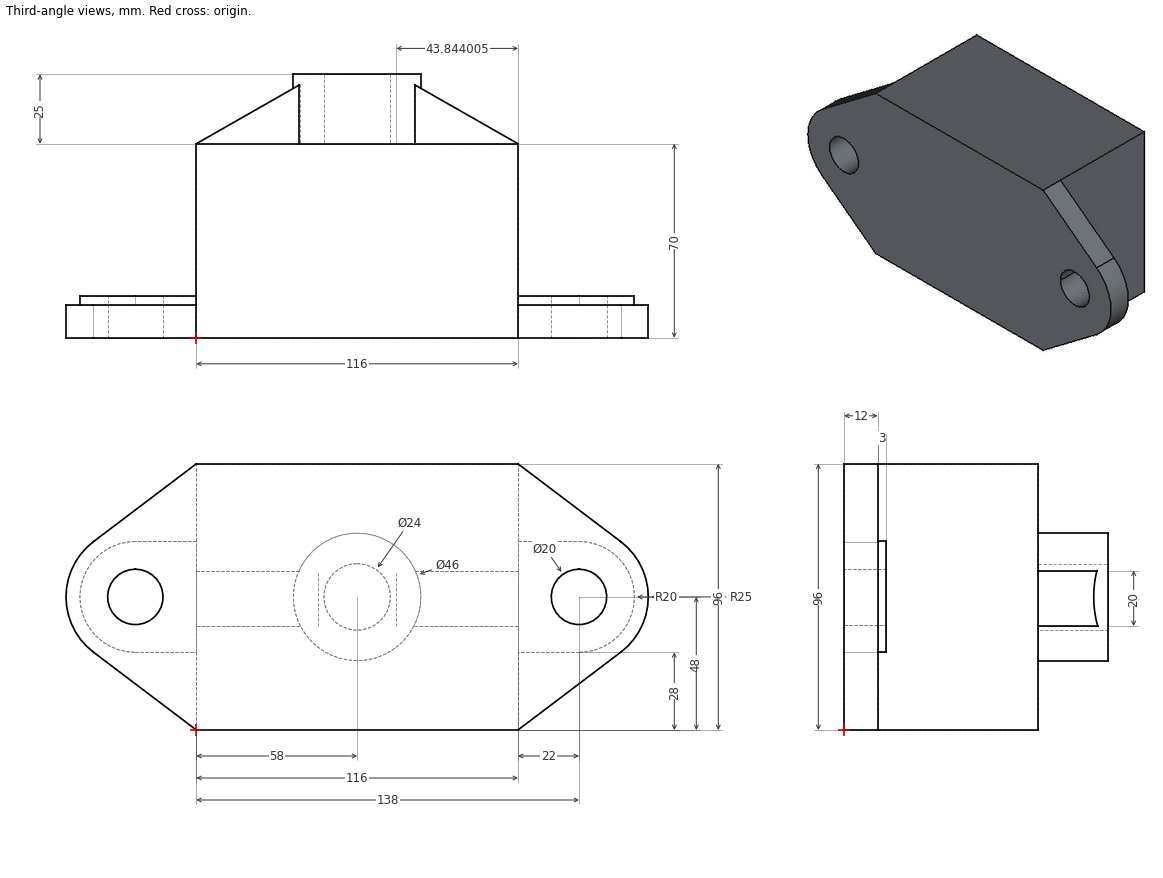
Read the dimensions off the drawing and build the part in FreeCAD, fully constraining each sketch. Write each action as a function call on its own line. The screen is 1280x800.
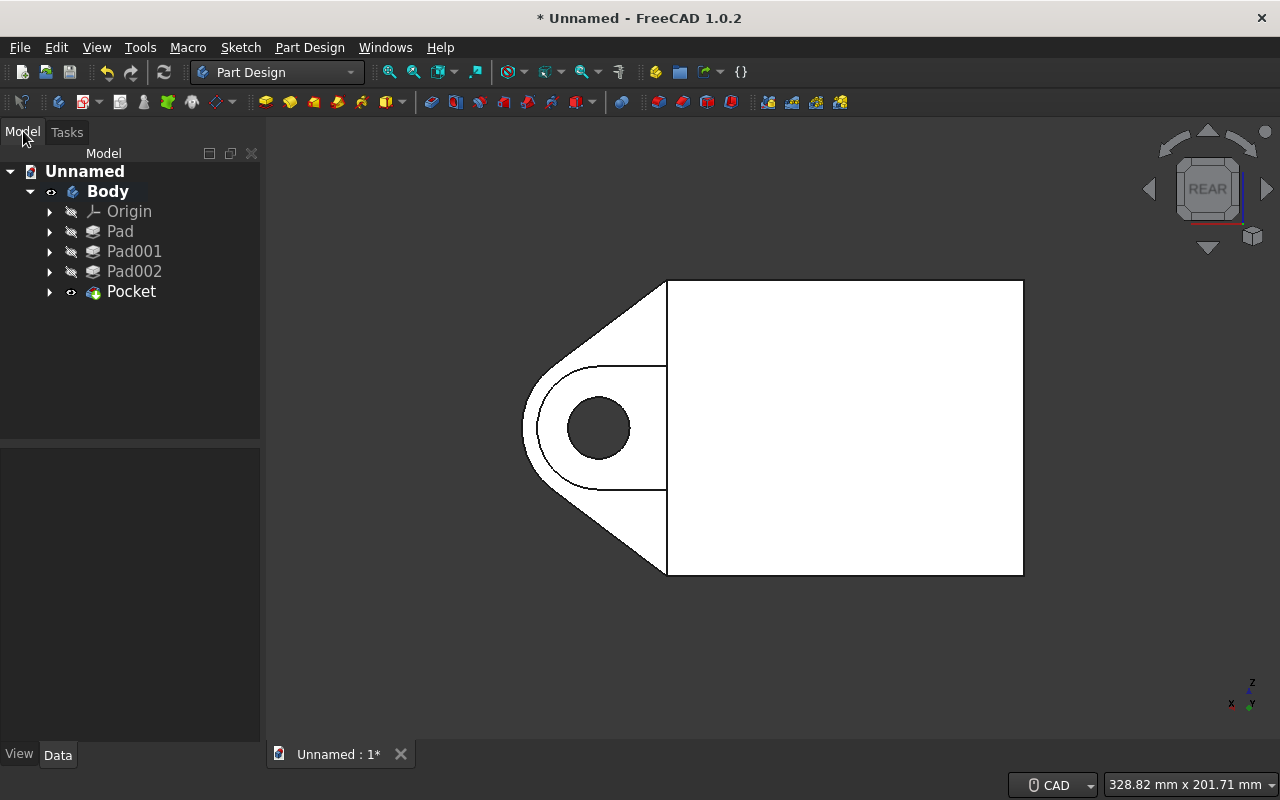
click(50, 212)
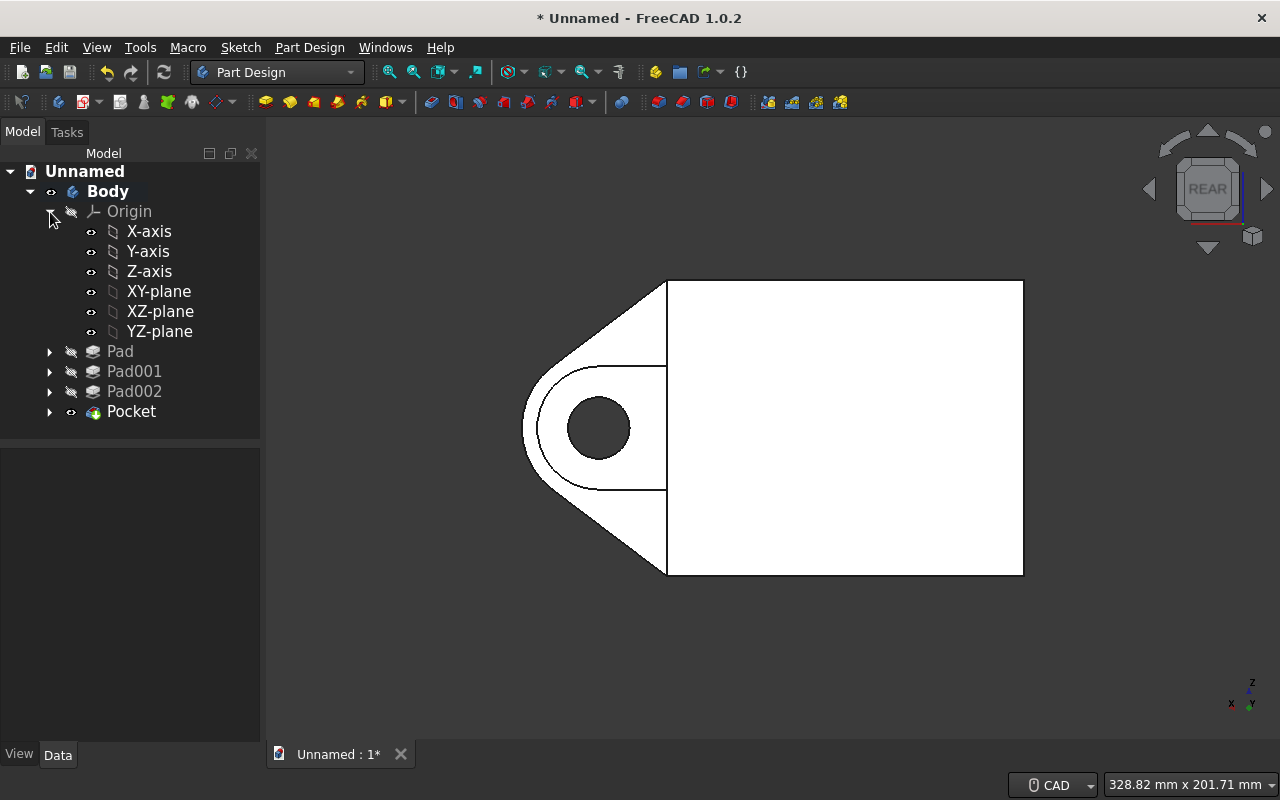
click(136, 332)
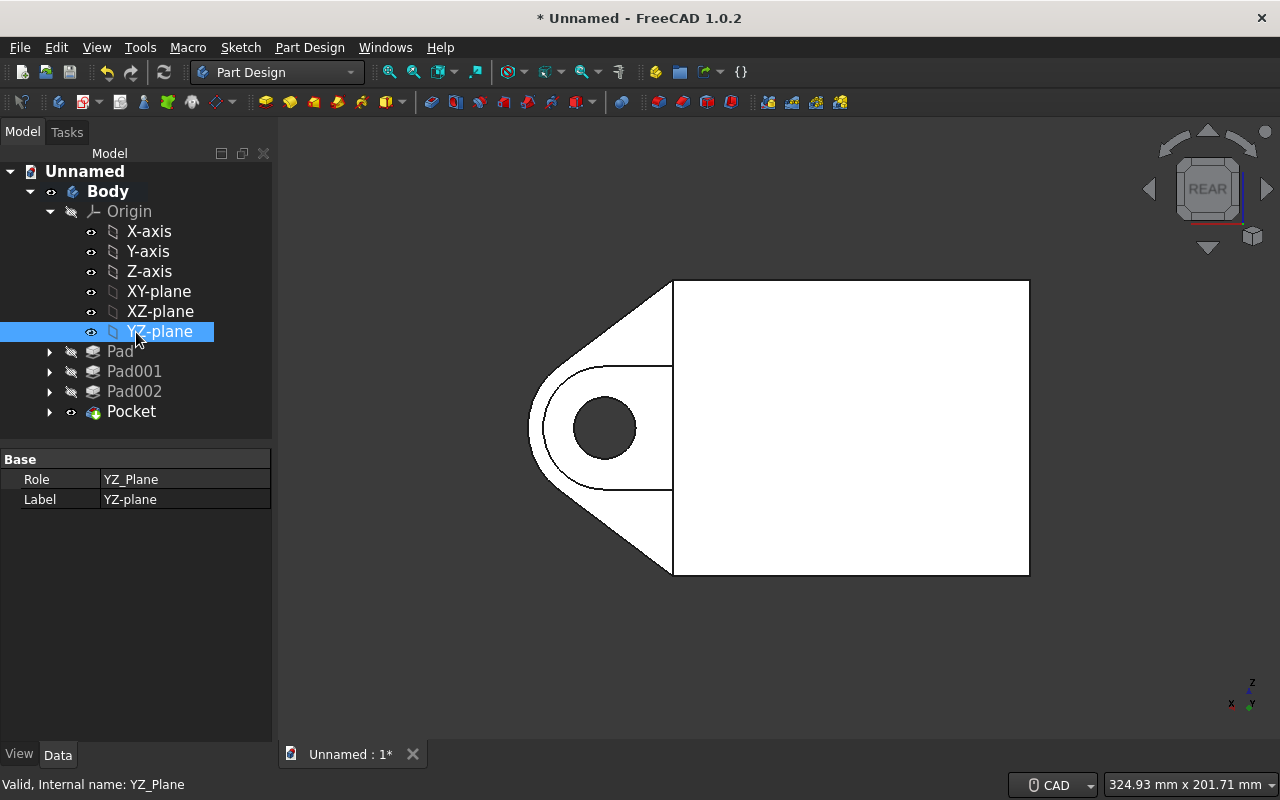
click(216, 102)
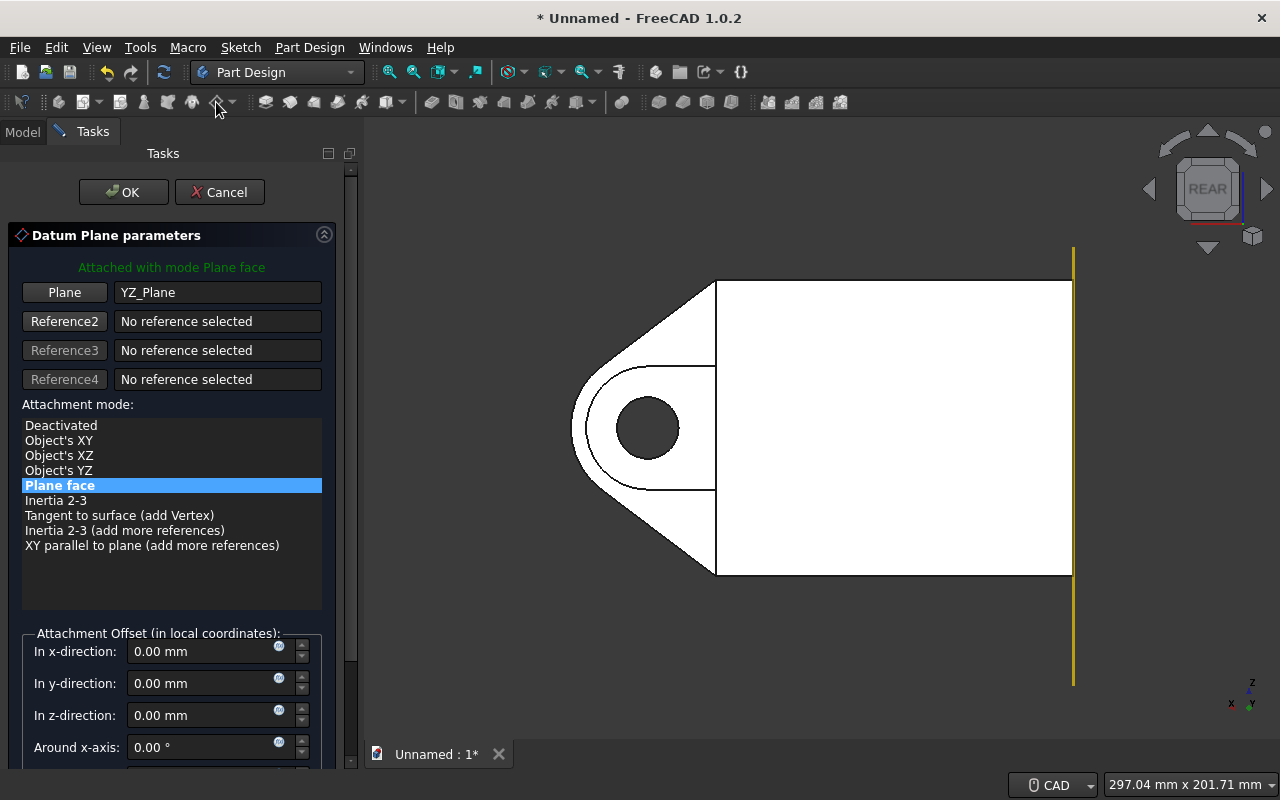
triple_click(210, 715)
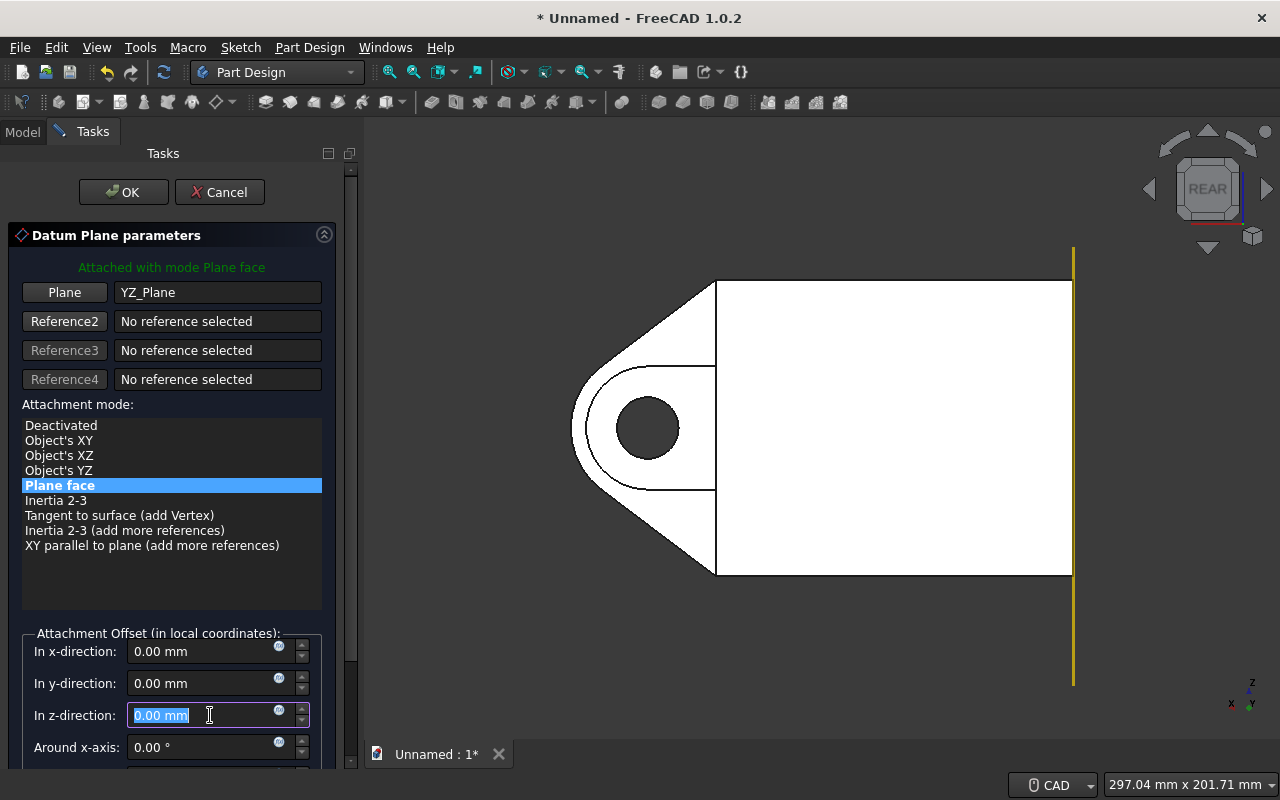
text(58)
key(Tab)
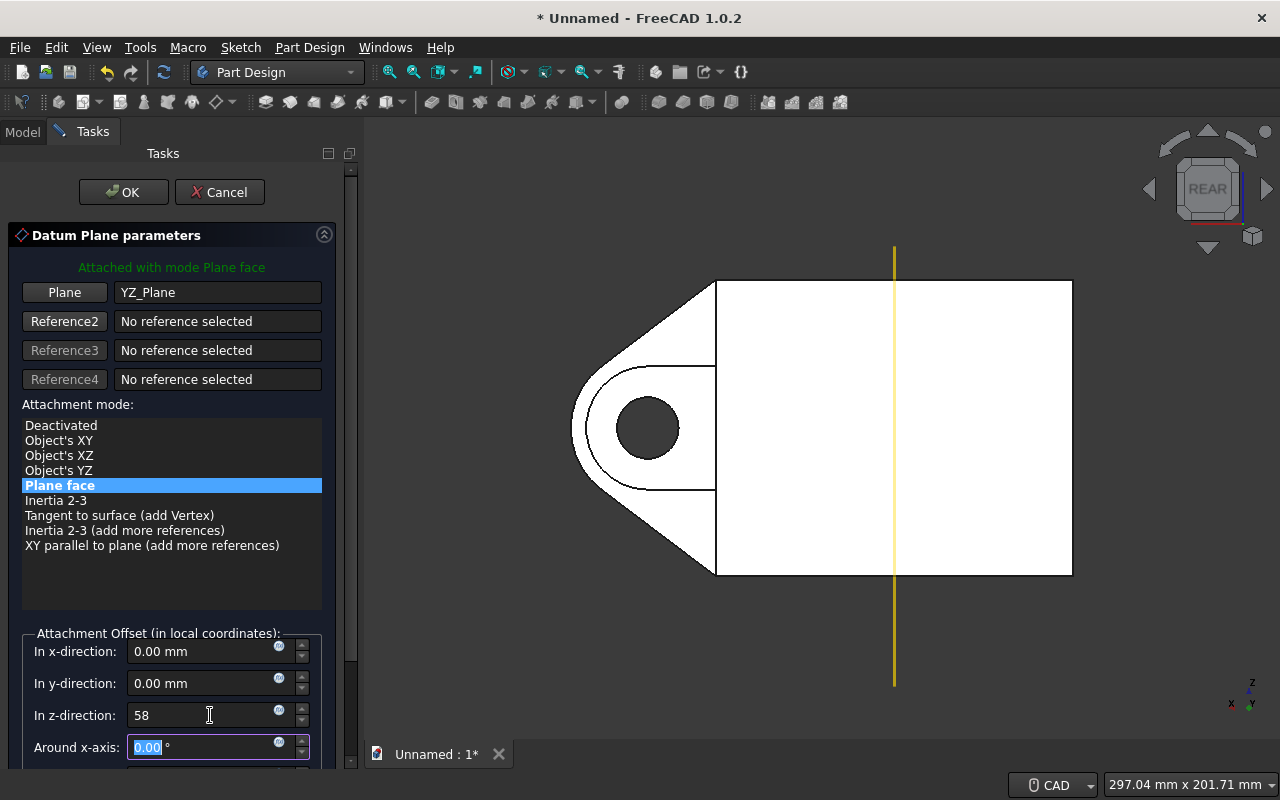
click(124, 192)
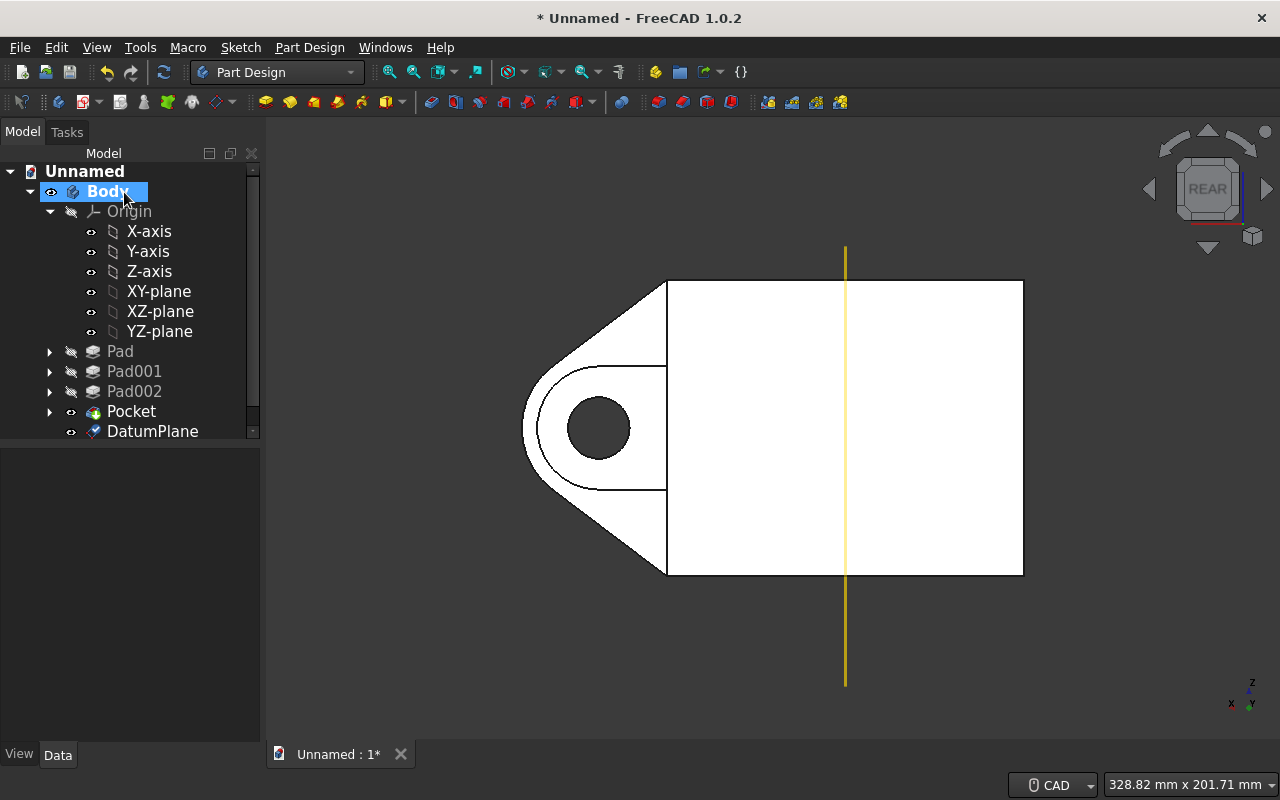
click(116, 372)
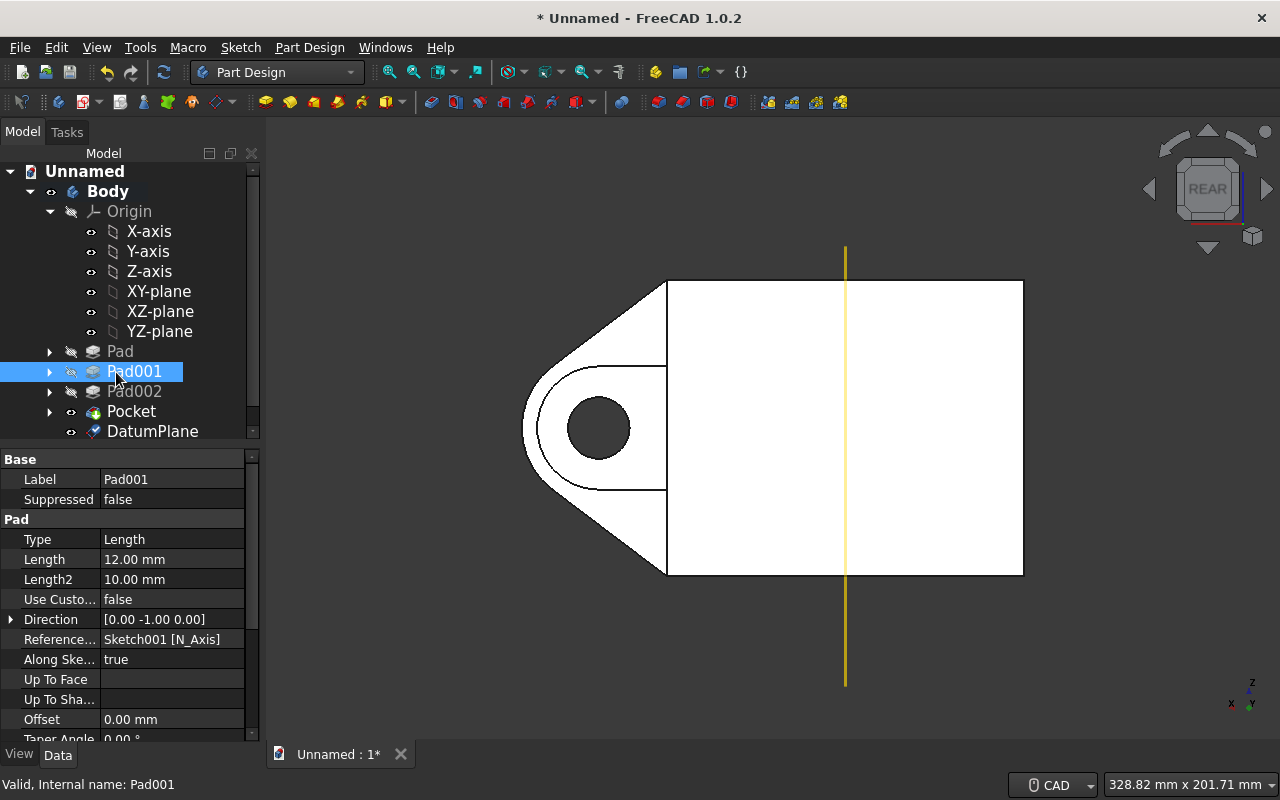
click(116, 392, ctrl)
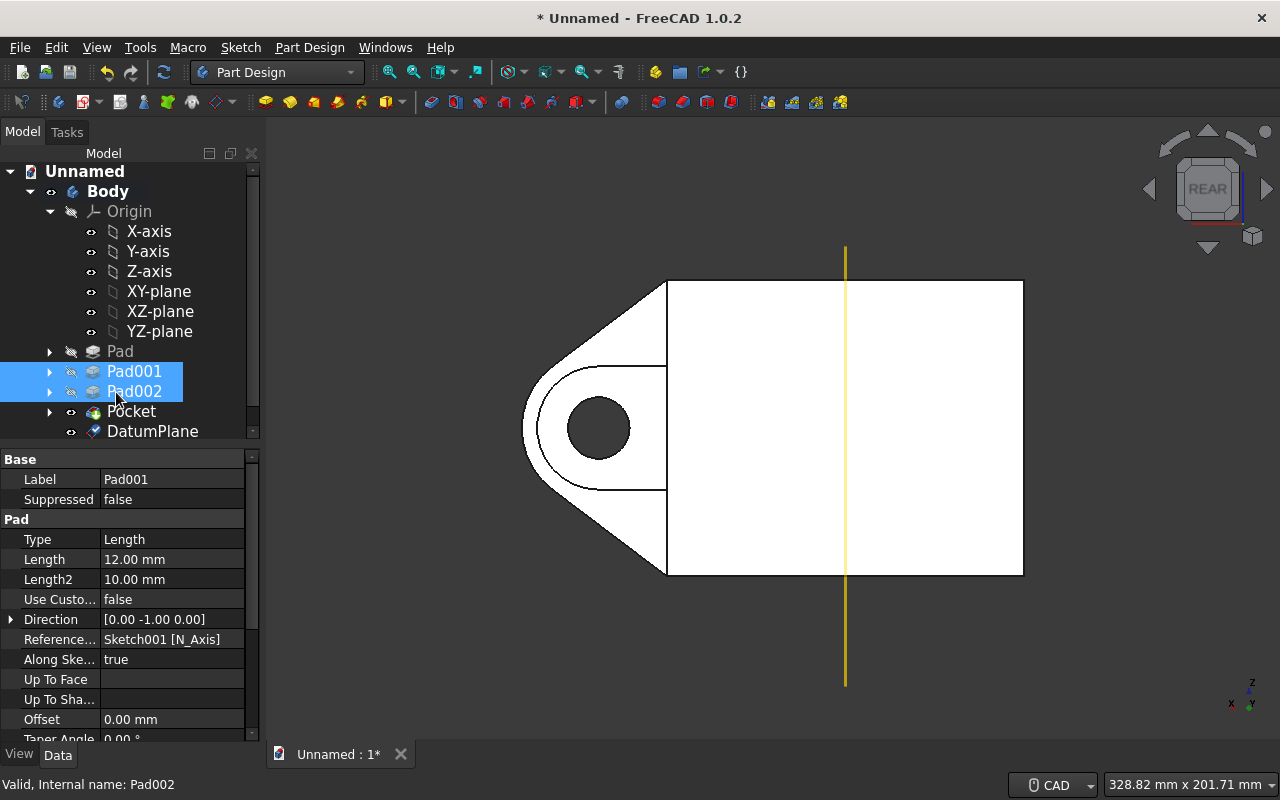
click(116, 412, ctrl)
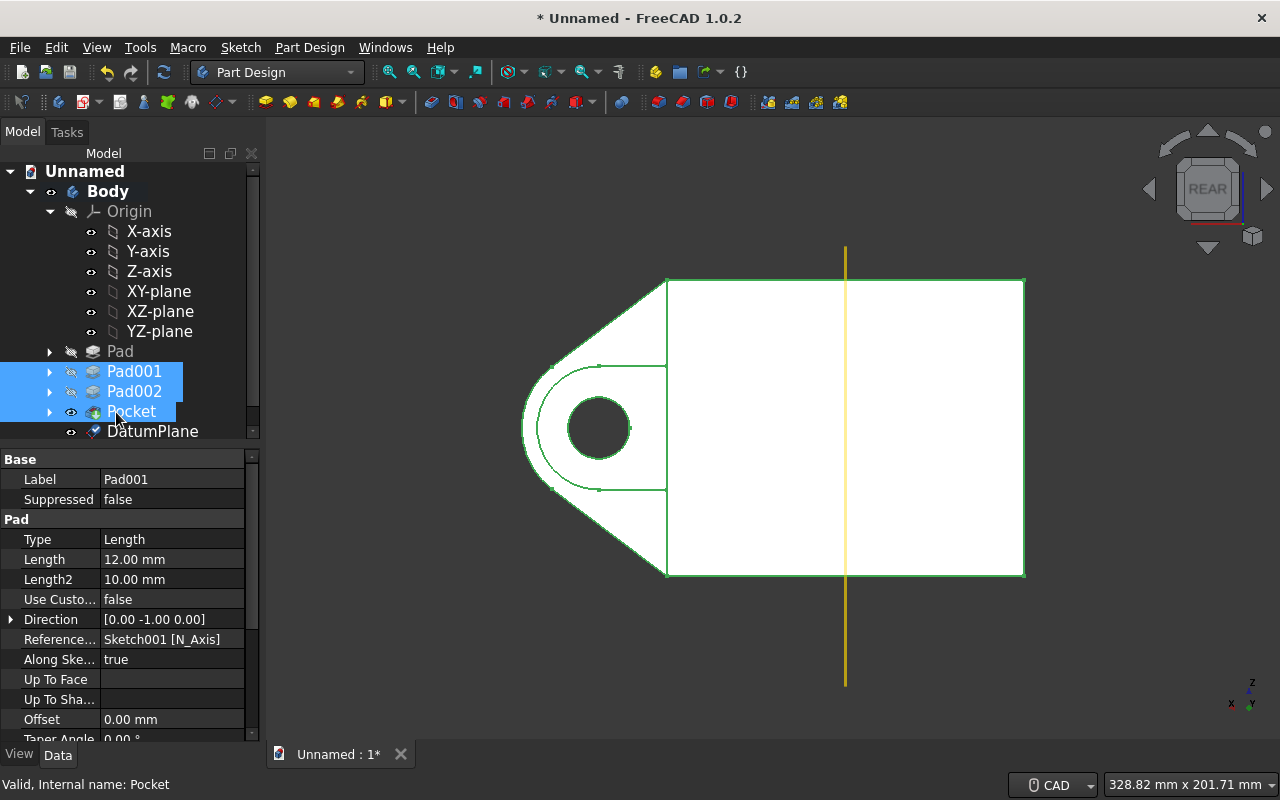
click(768, 102)